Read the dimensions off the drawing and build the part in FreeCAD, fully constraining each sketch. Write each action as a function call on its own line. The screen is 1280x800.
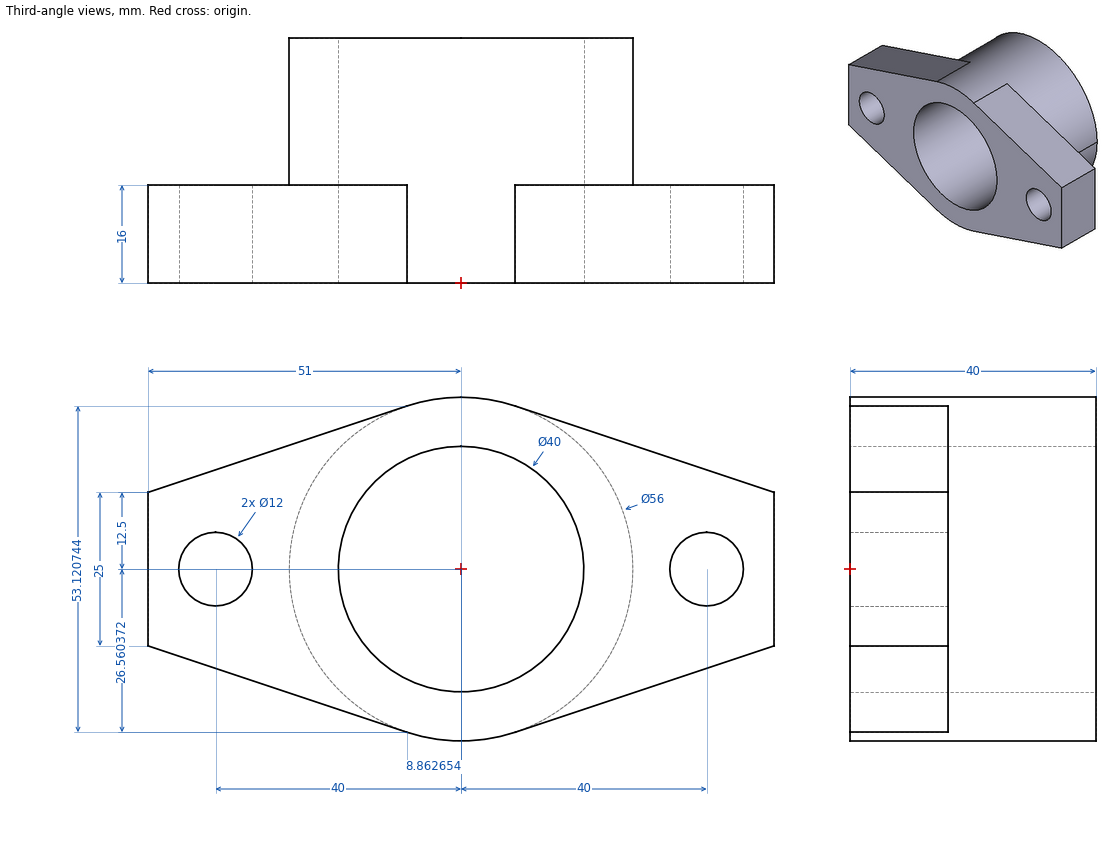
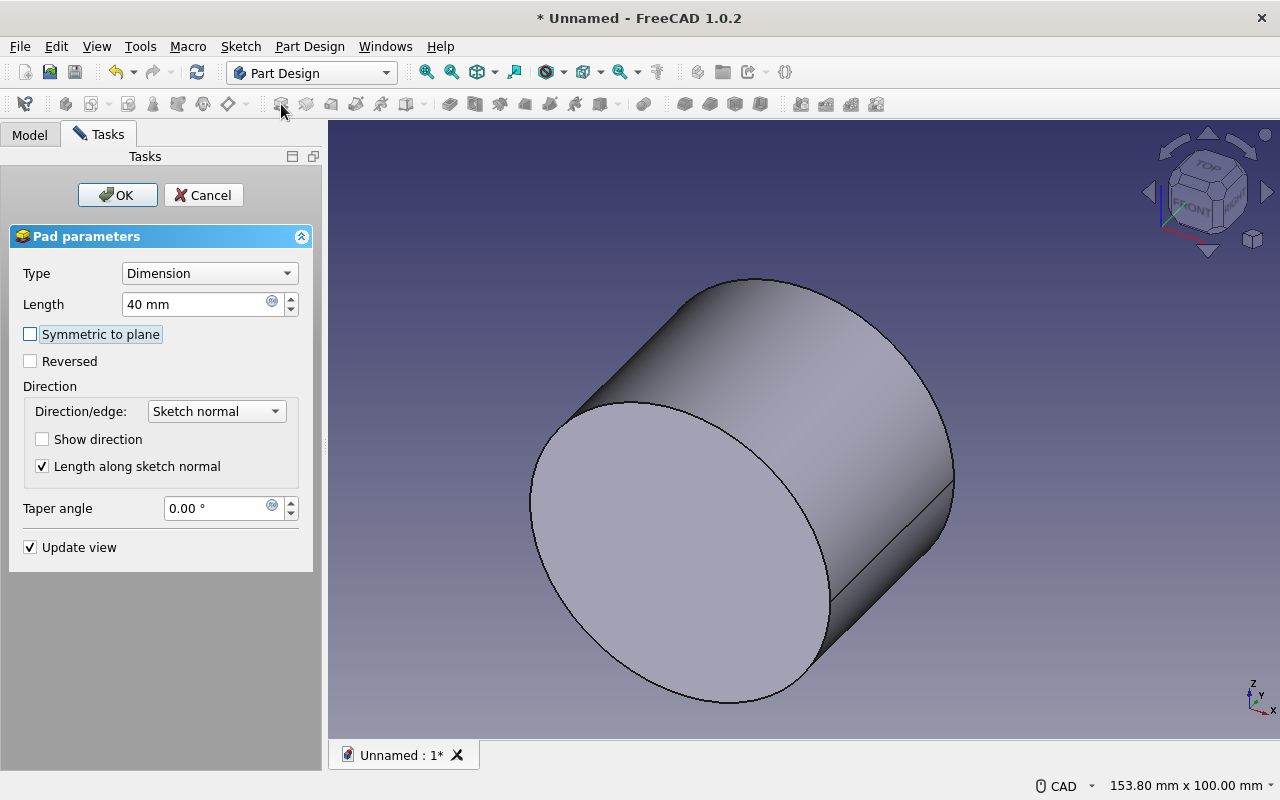
click(31, 361)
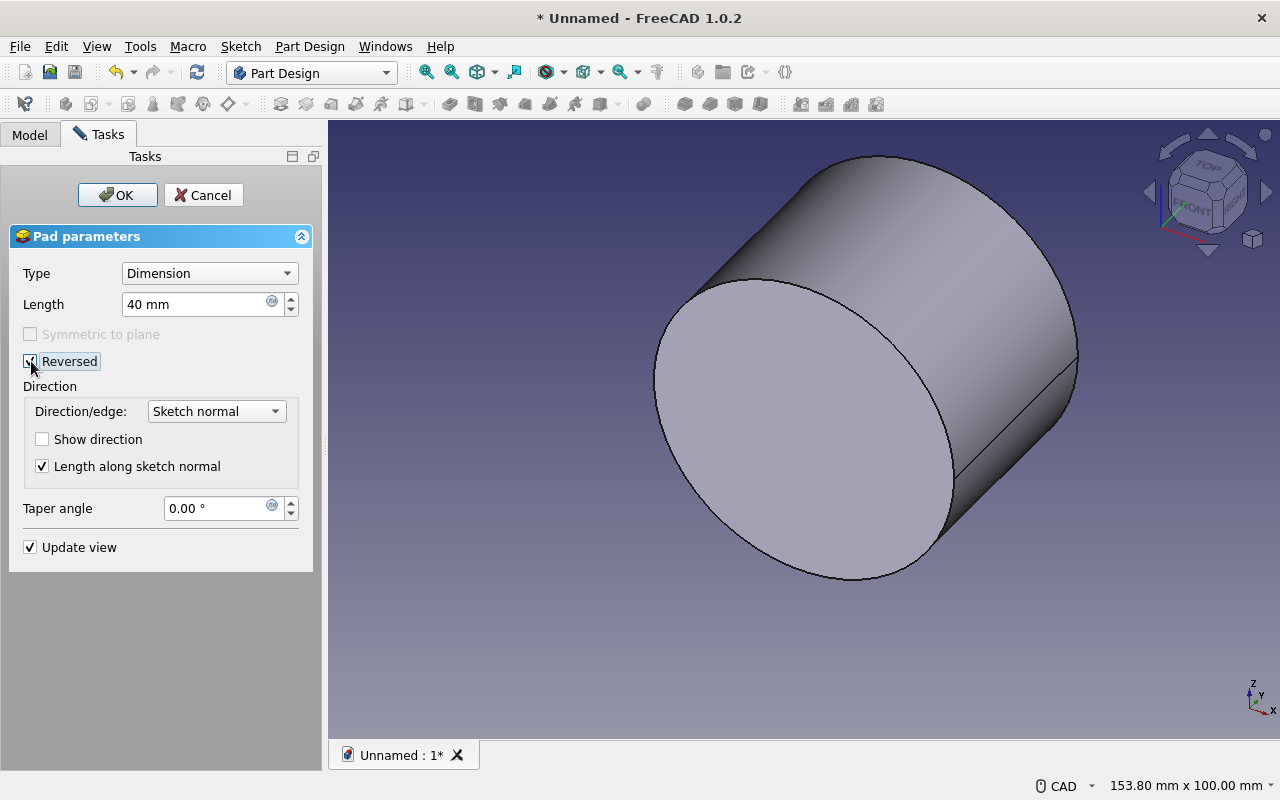
click(118, 195)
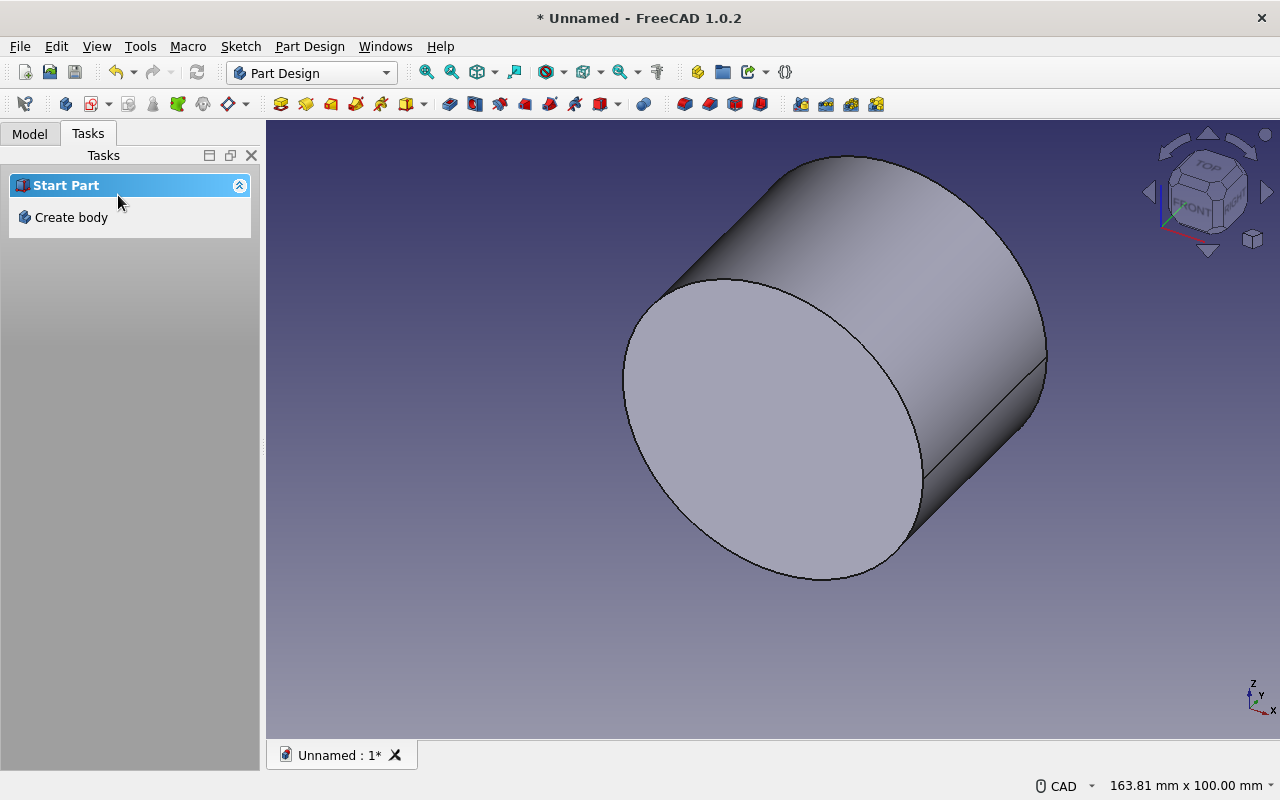
click(427, 72)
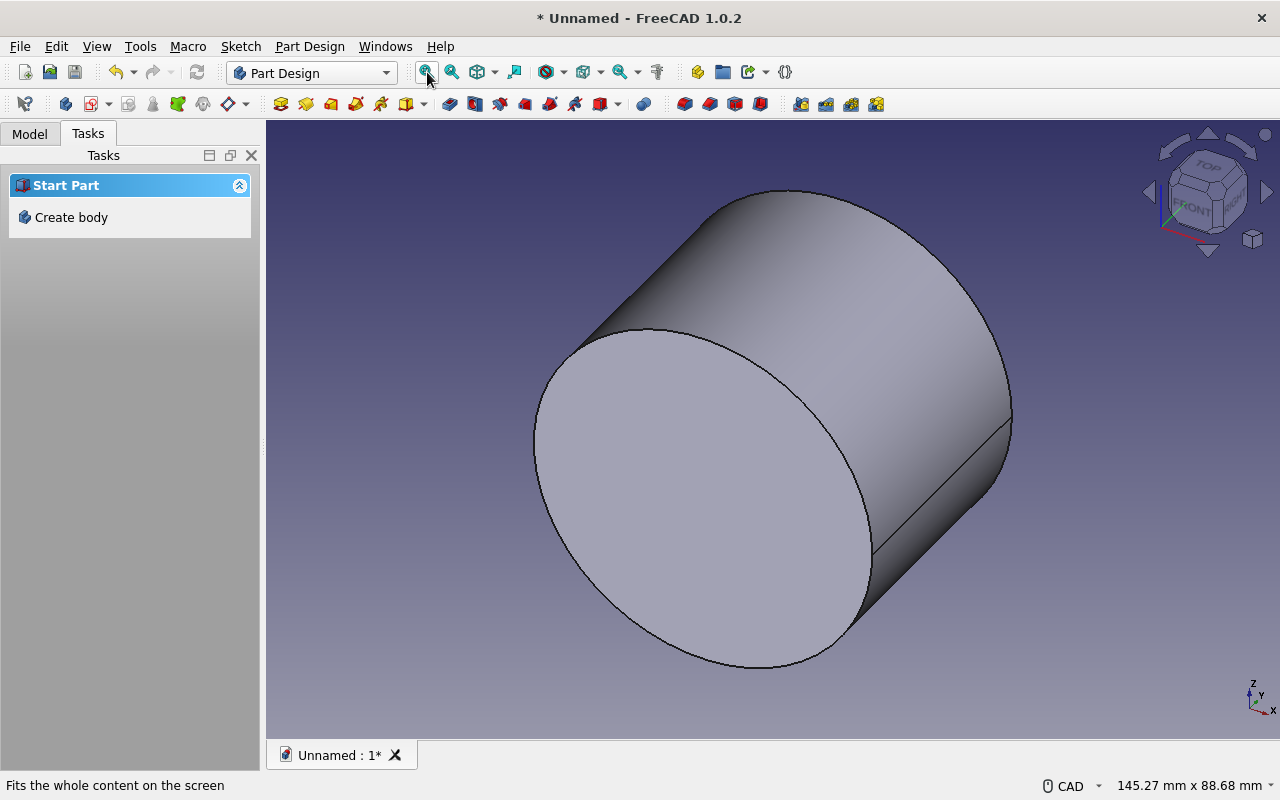
click(90, 104)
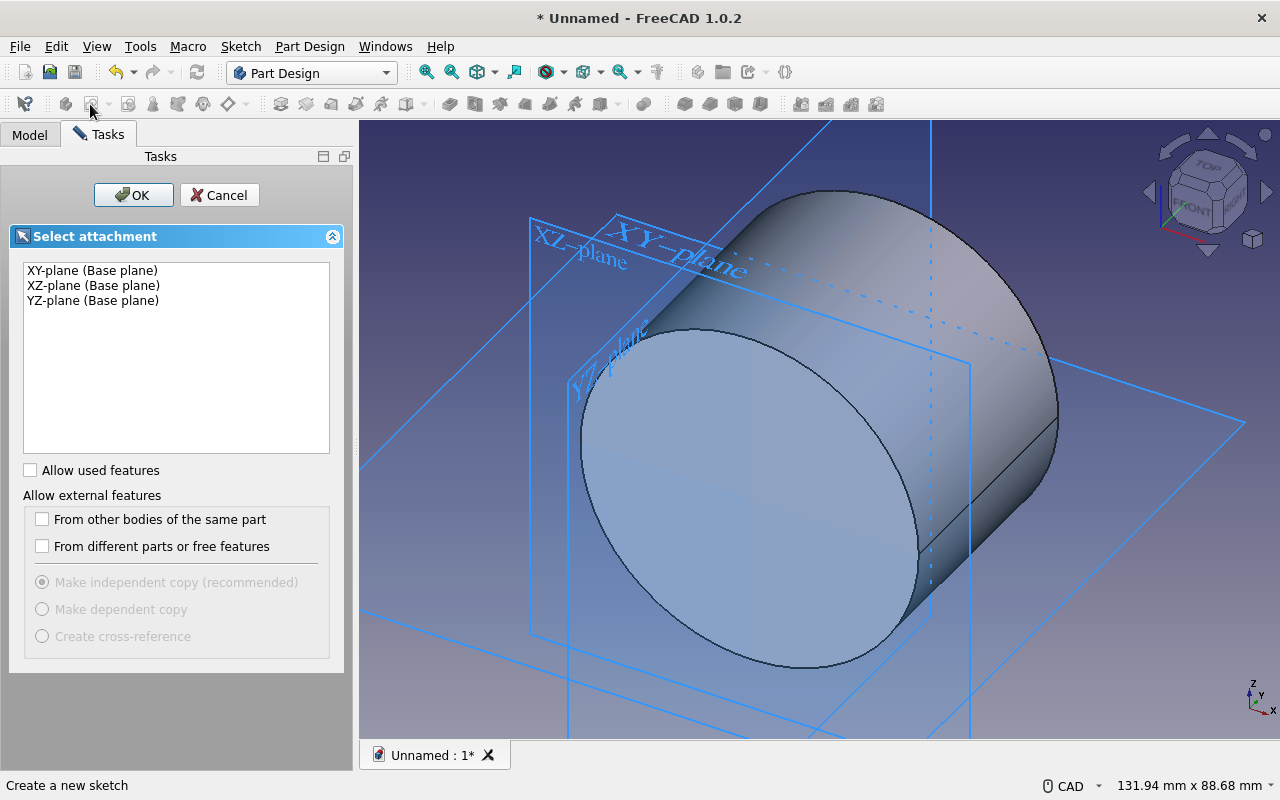
click(84, 286)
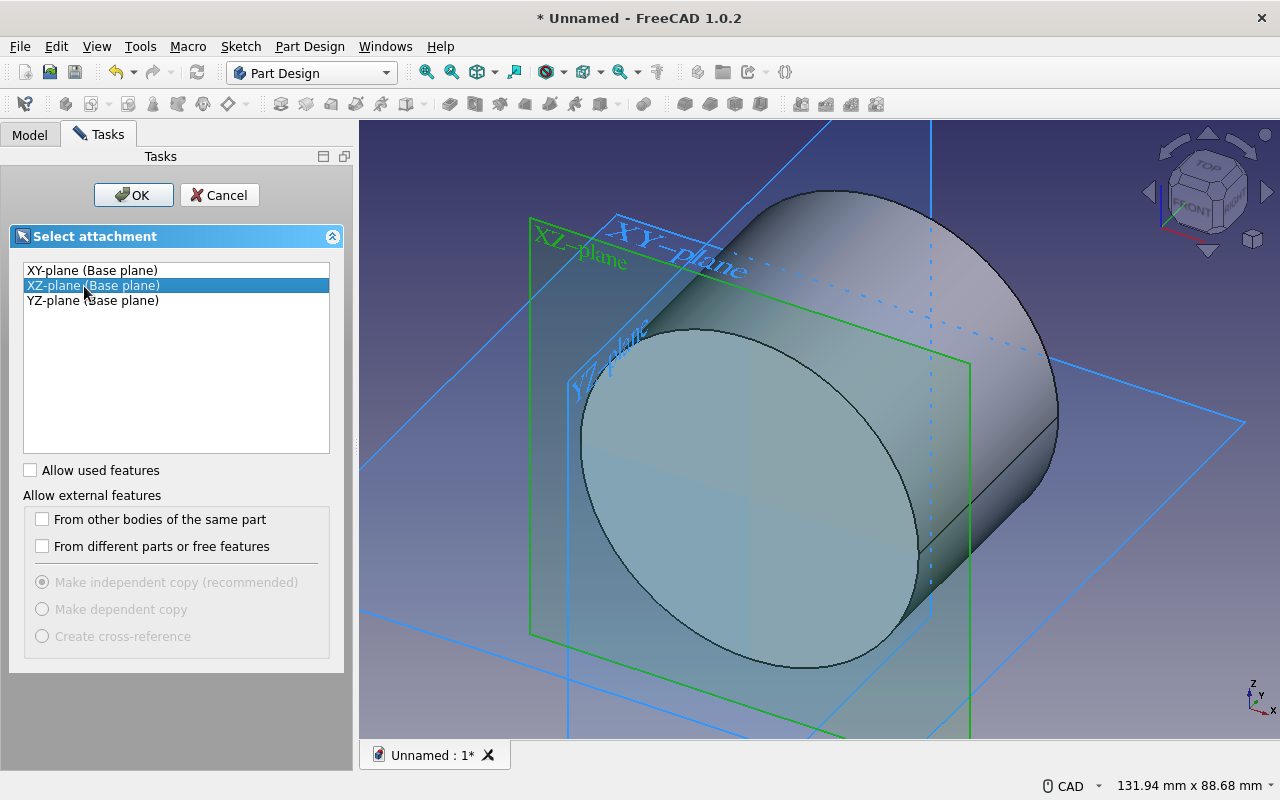
click(134, 195)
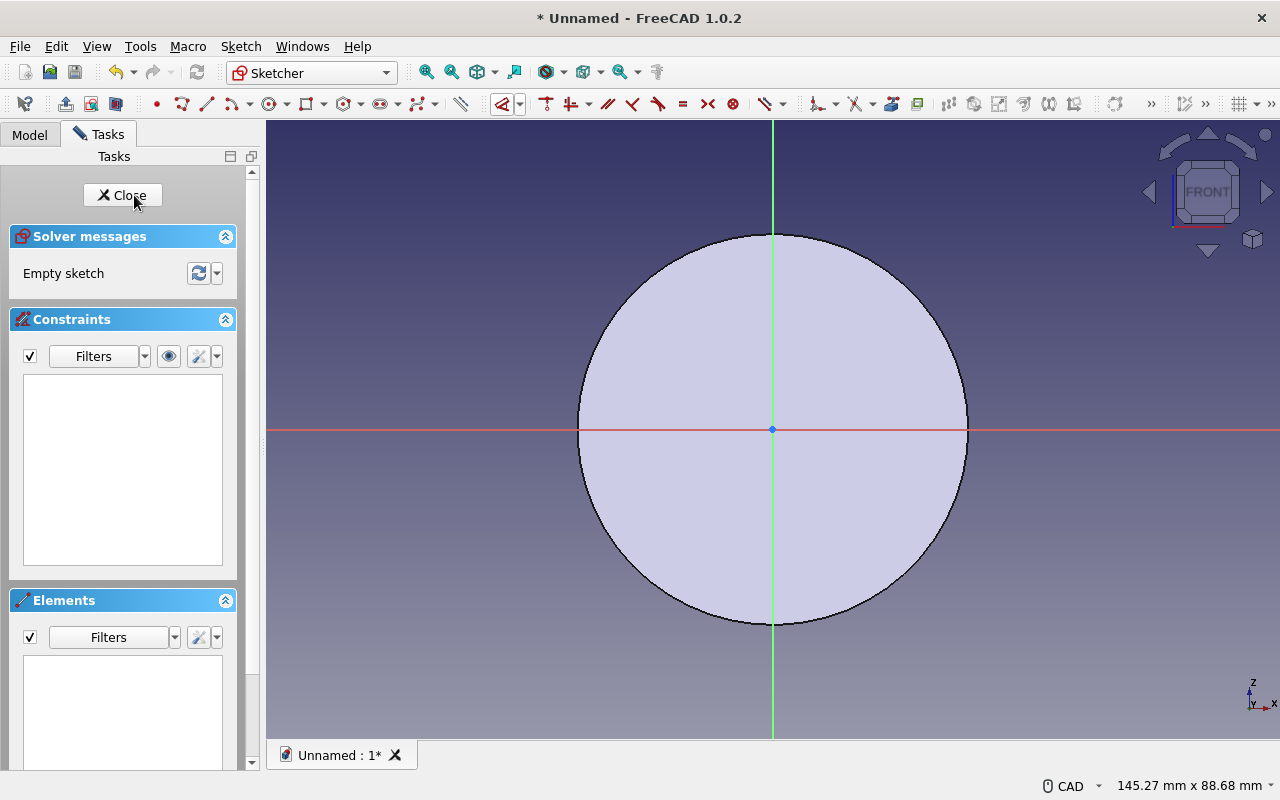
click(182, 104)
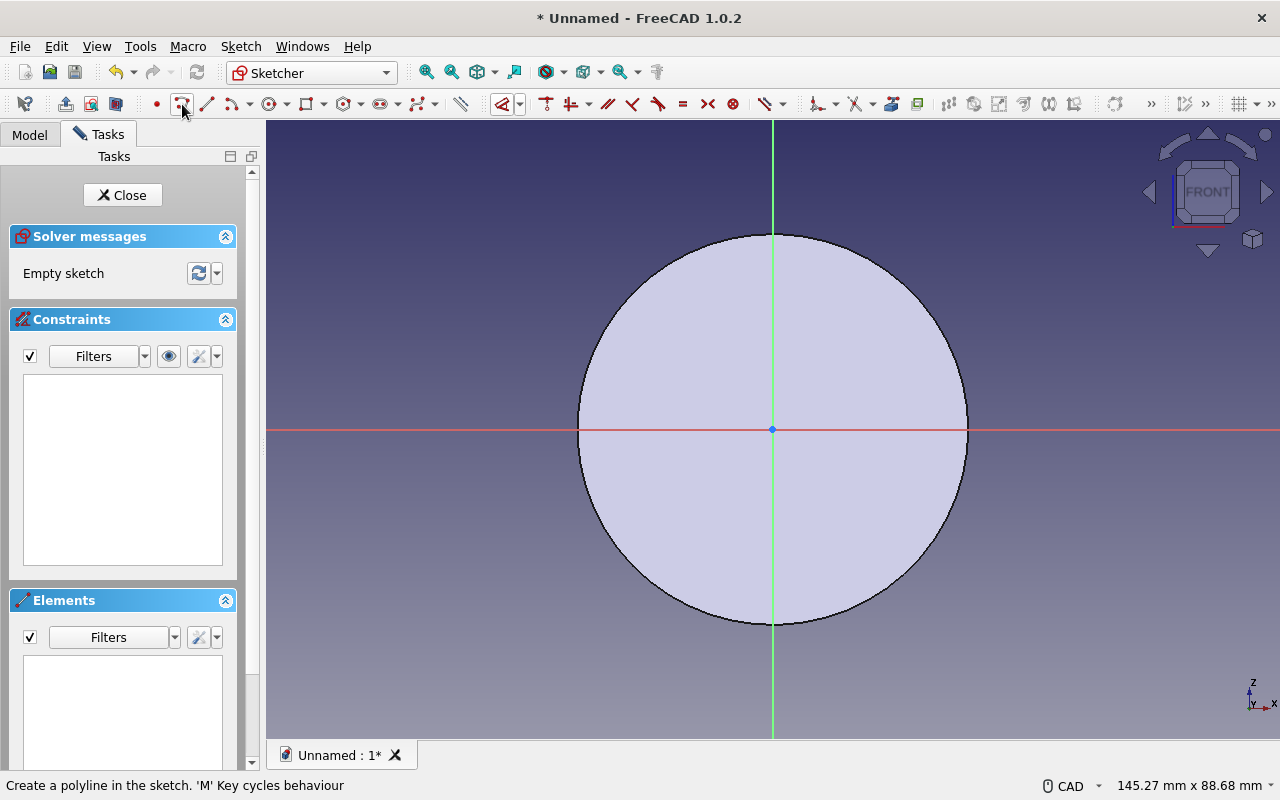
click(711, 615)
click(711, 244)
click(417, 342)
click(417, 517)
click(711, 616)
key(Escape)
key(Escape)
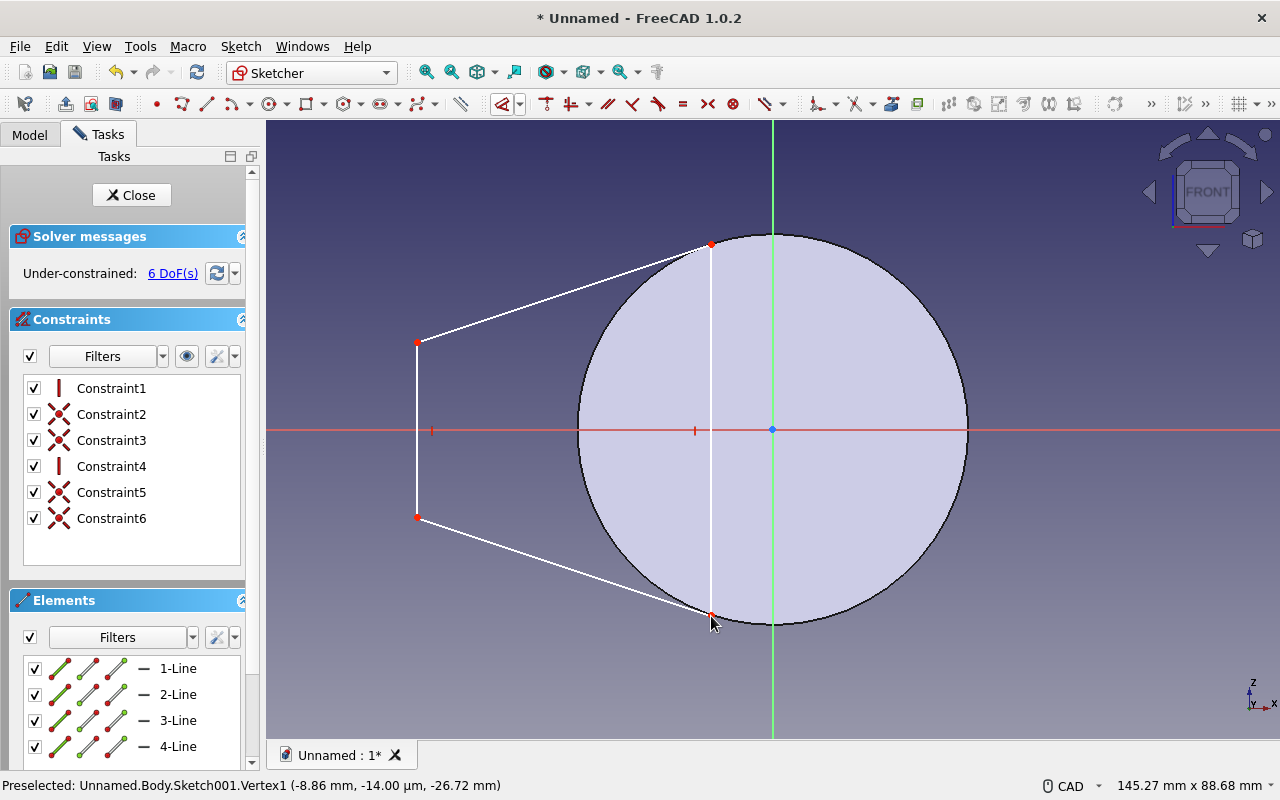
click(502, 104)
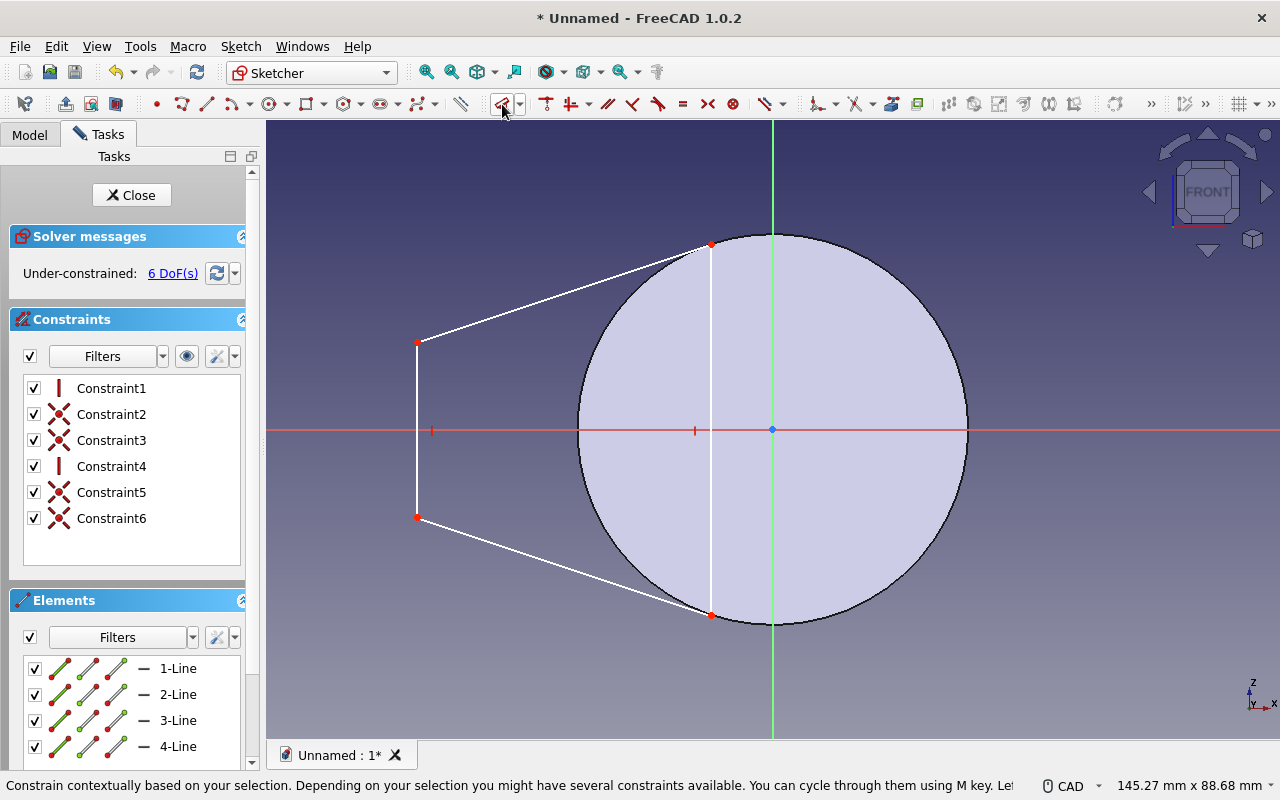
click(417, 395)
click(383, 390)